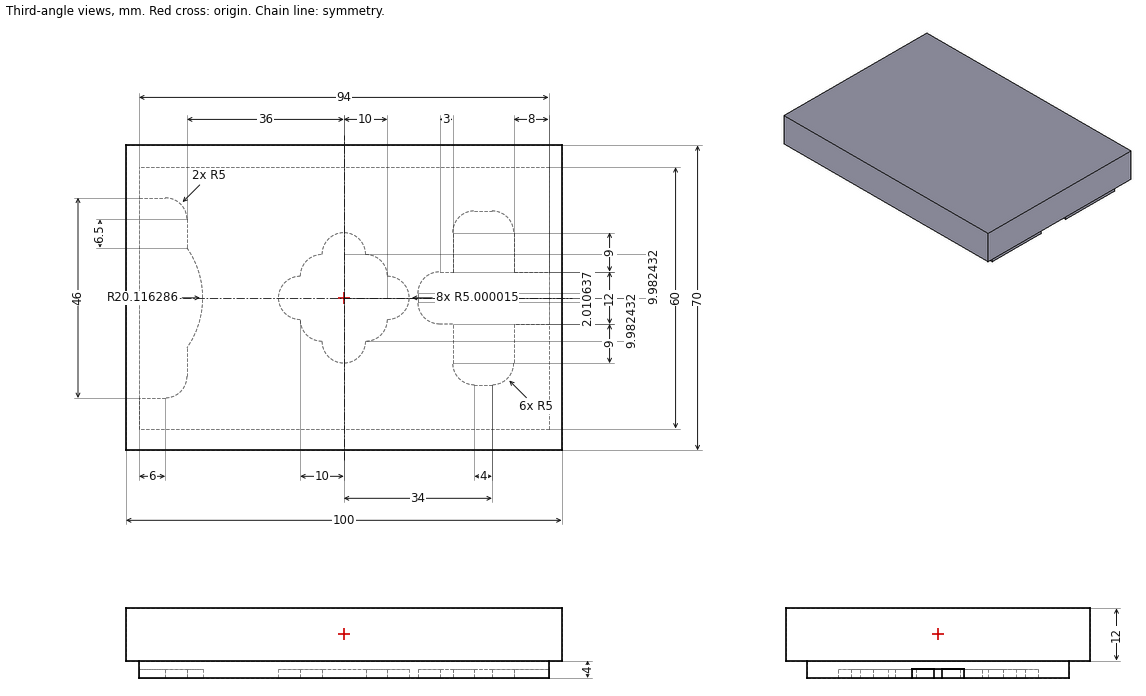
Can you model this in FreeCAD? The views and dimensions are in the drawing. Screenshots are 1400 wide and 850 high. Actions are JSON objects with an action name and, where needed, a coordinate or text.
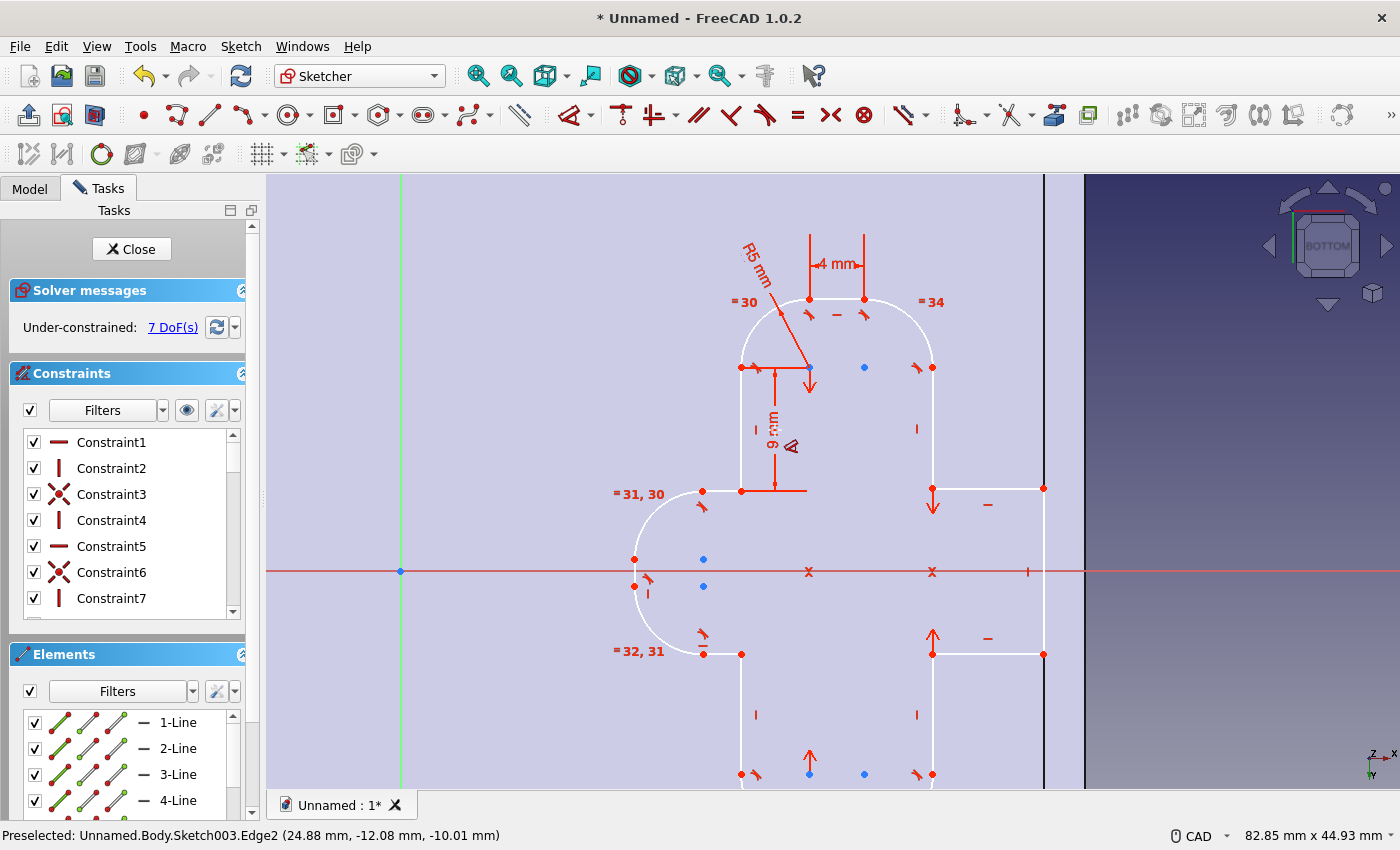
{"action": "left_click", "coordinate": [715, 654]}
{"action": "left_click", "coordinate": [722, 688]}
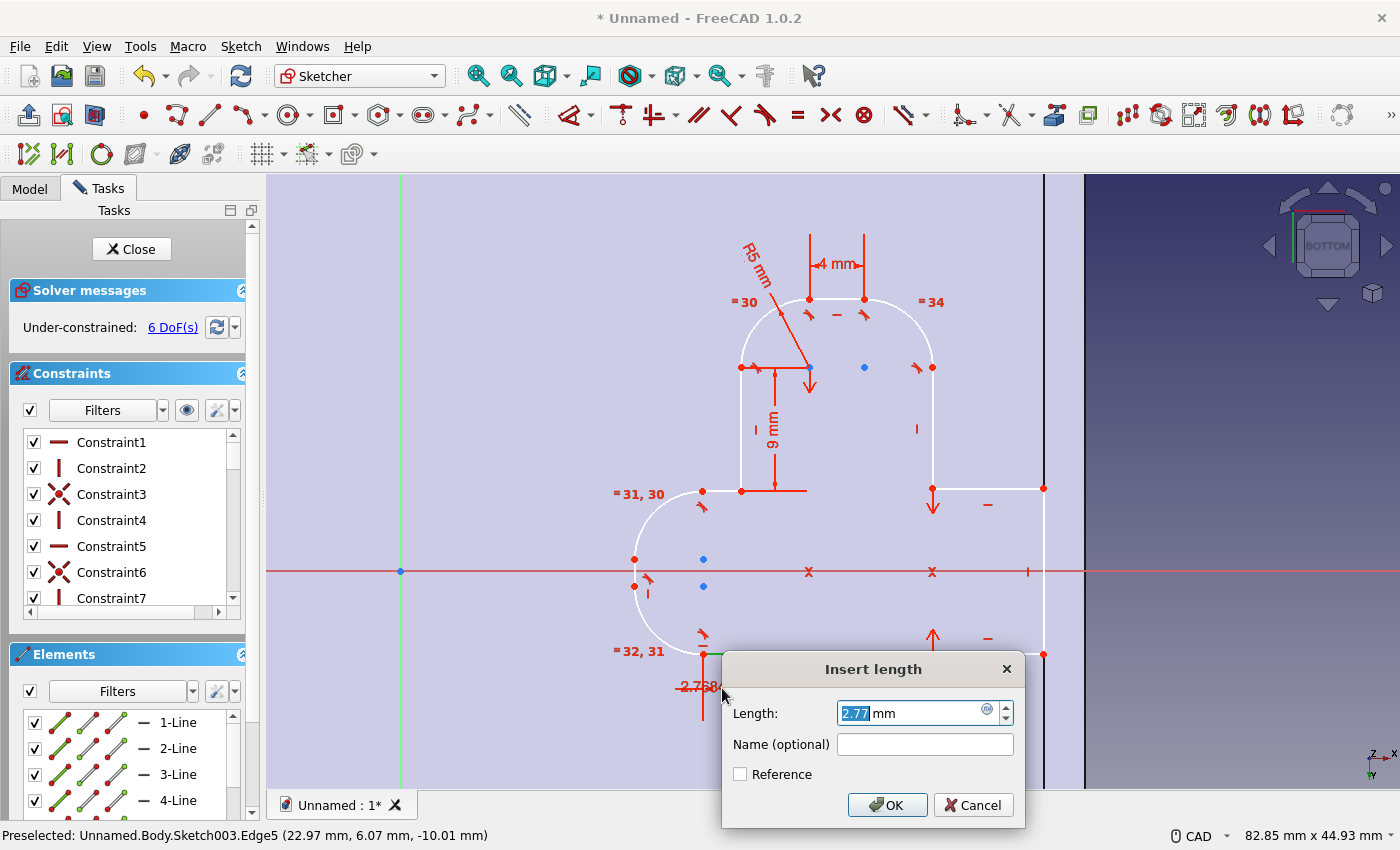
{"action": "type", "text": "3"}
{"action": "key", "text": "Return"}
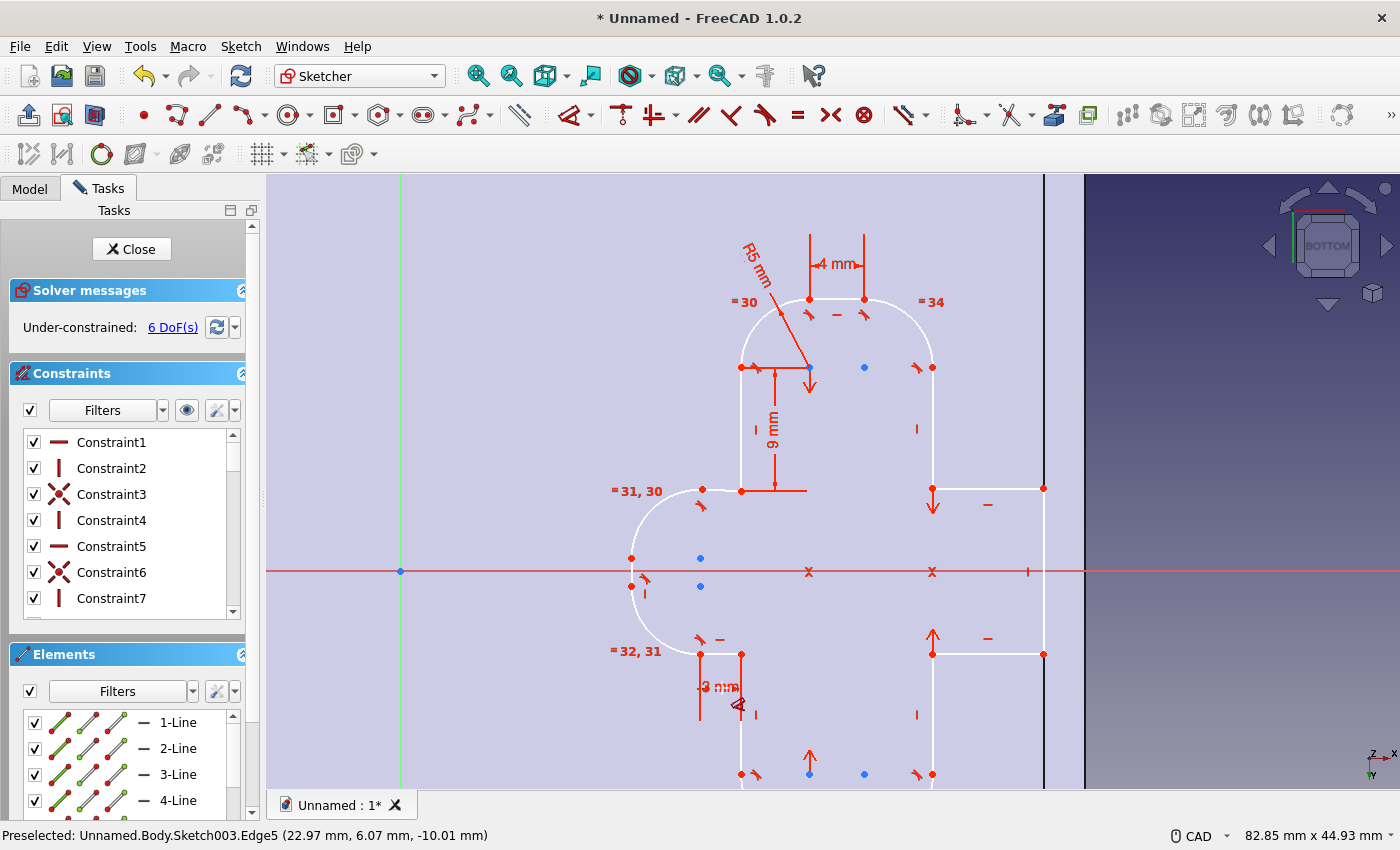
{"action": "left_click", "coordinate": [741, 691]}
{"action": "left_click", "coordinate": [775, 732]}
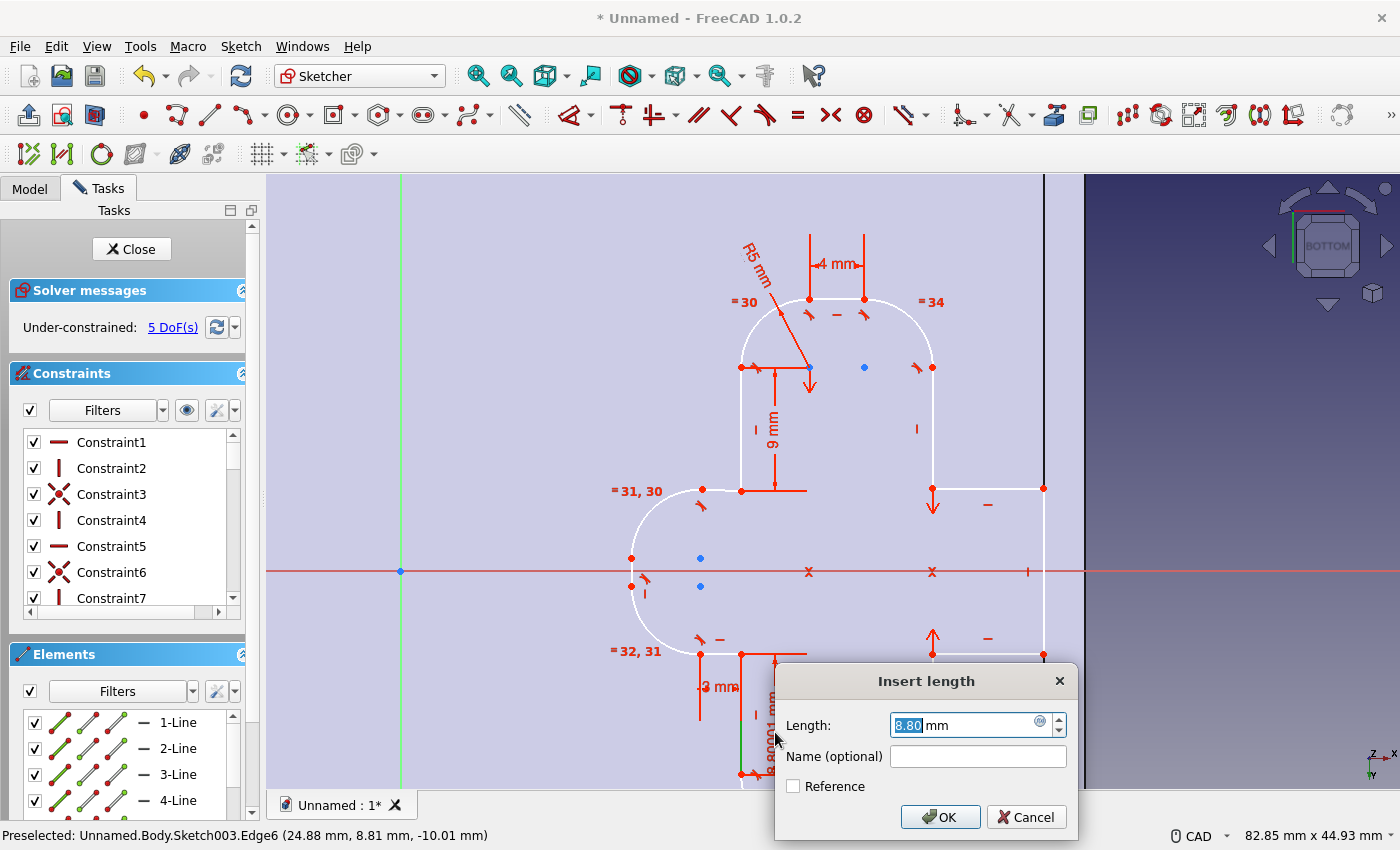
{"action": "type", "text": "9"}
{"action": "key", "text": "Return"}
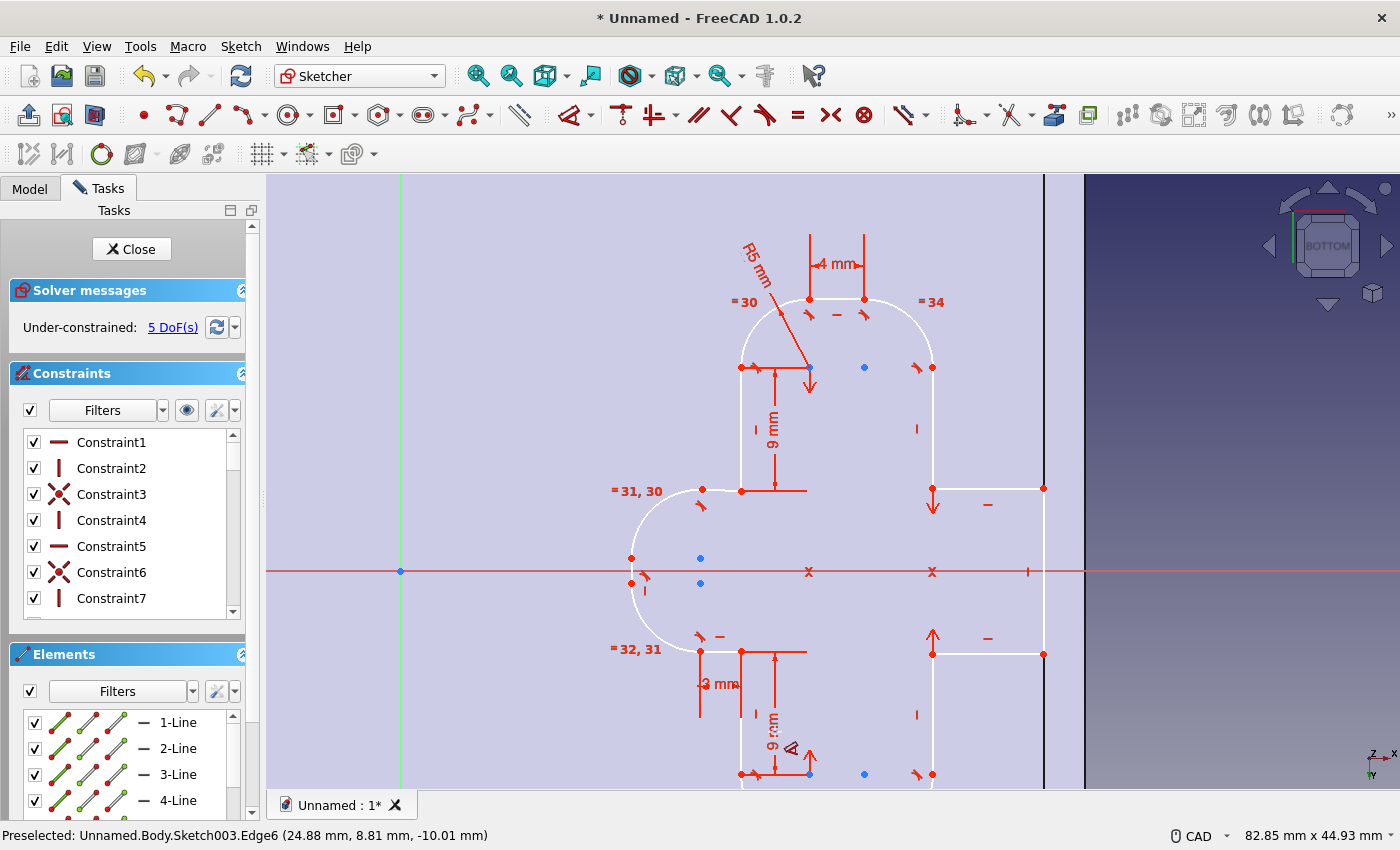
{"action": "left_click", "coordinate": [933, 739]}
{"action": "left_click", "coordinate": [967, 708]}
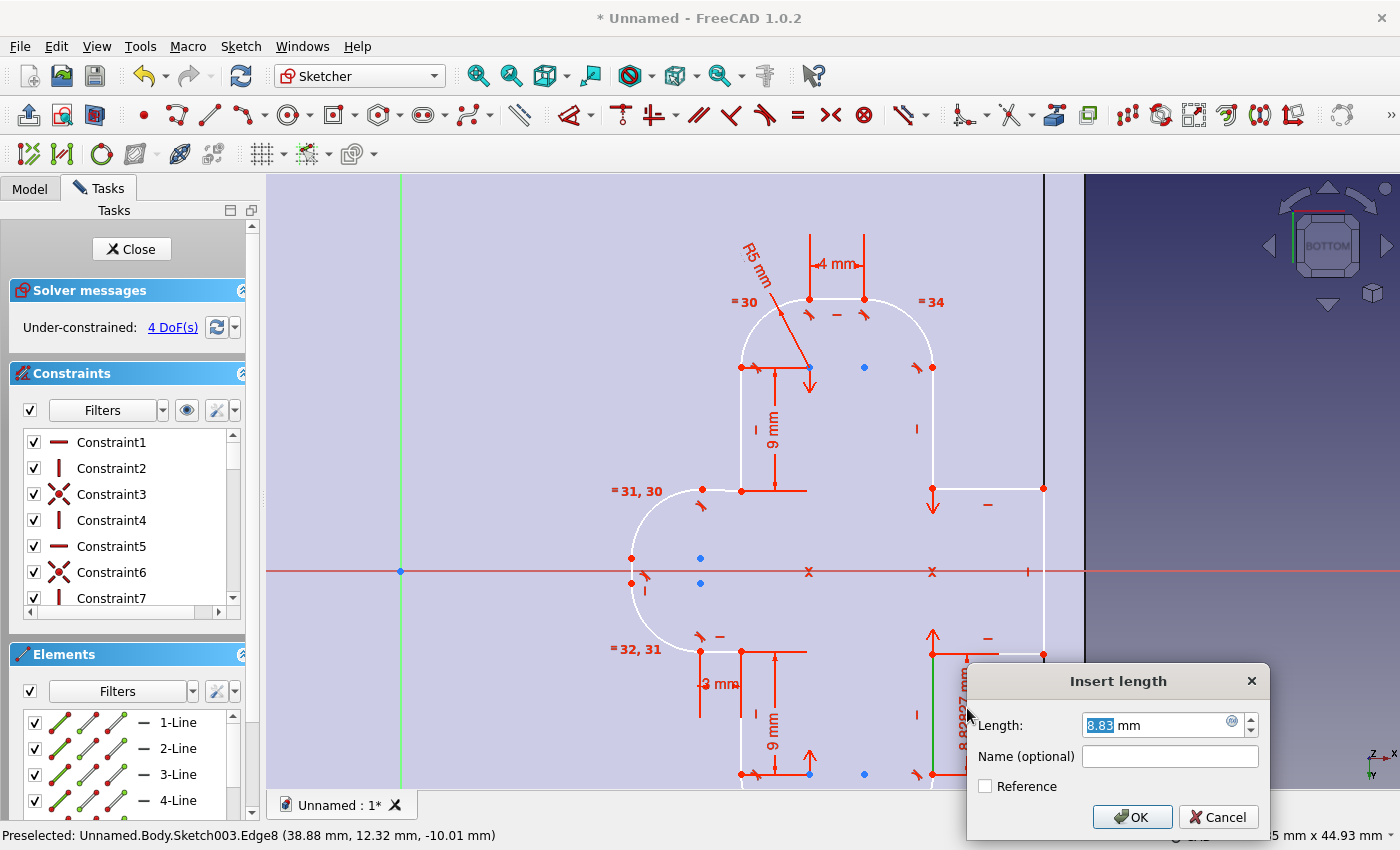
{"action": "type", "text": "9"}
{"action": "key", "text": "Return"}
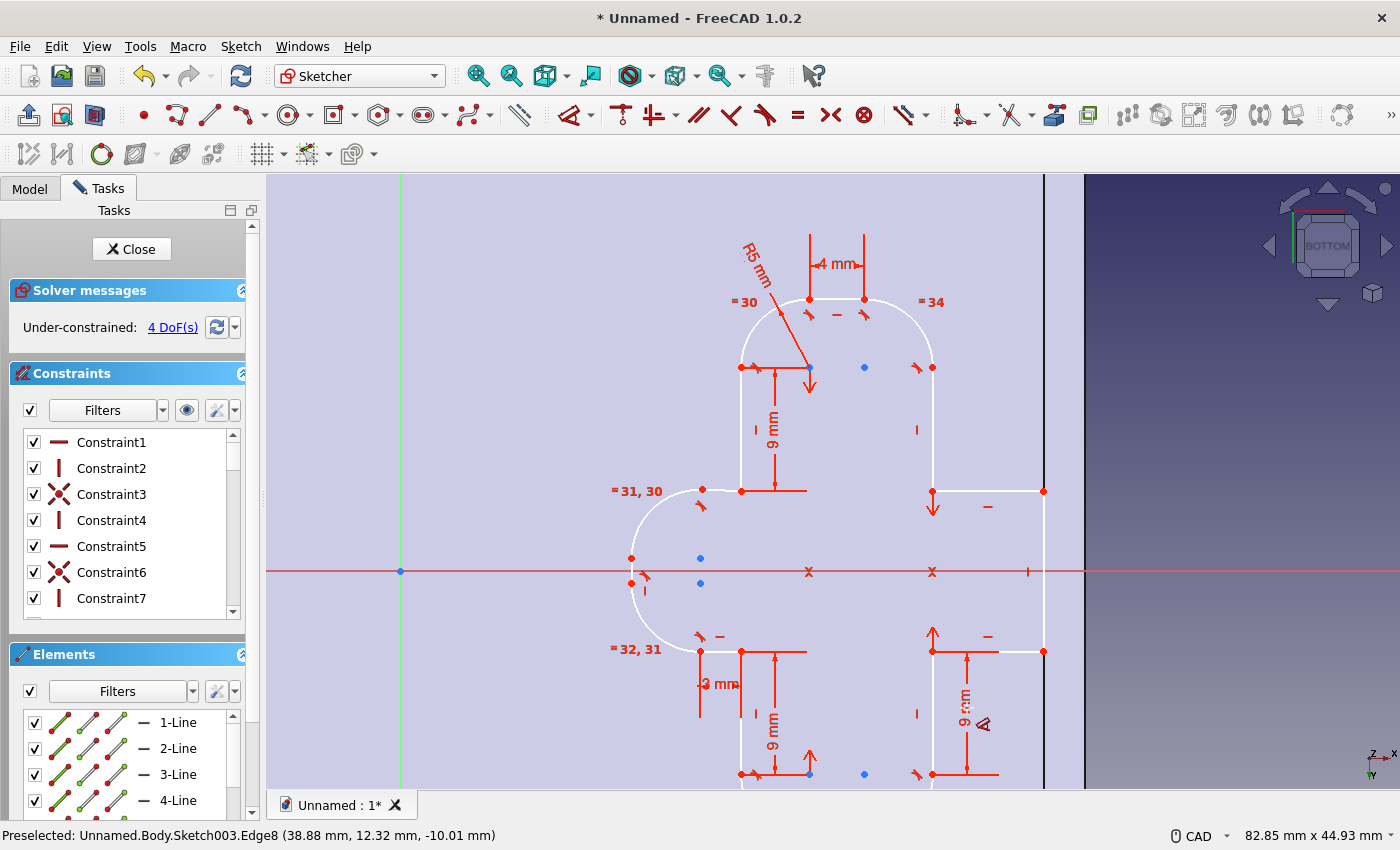
{"action": "left_click", "coordinate": [966, 652]}
{"action": "left_click", "coordinate": [988, 686]}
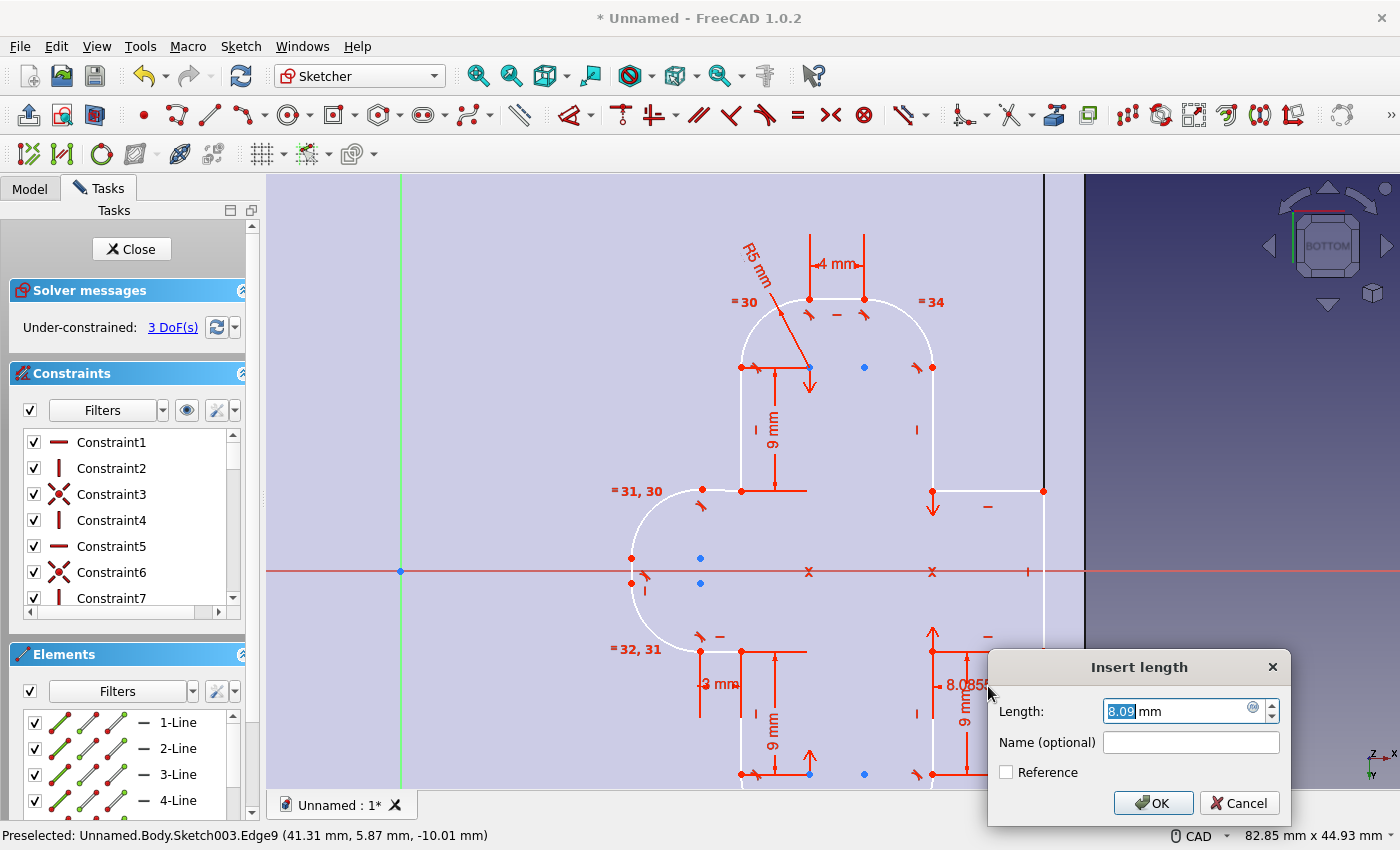
{"action": "type", "text": "8"}
{"action": "key", "text": "Return"}